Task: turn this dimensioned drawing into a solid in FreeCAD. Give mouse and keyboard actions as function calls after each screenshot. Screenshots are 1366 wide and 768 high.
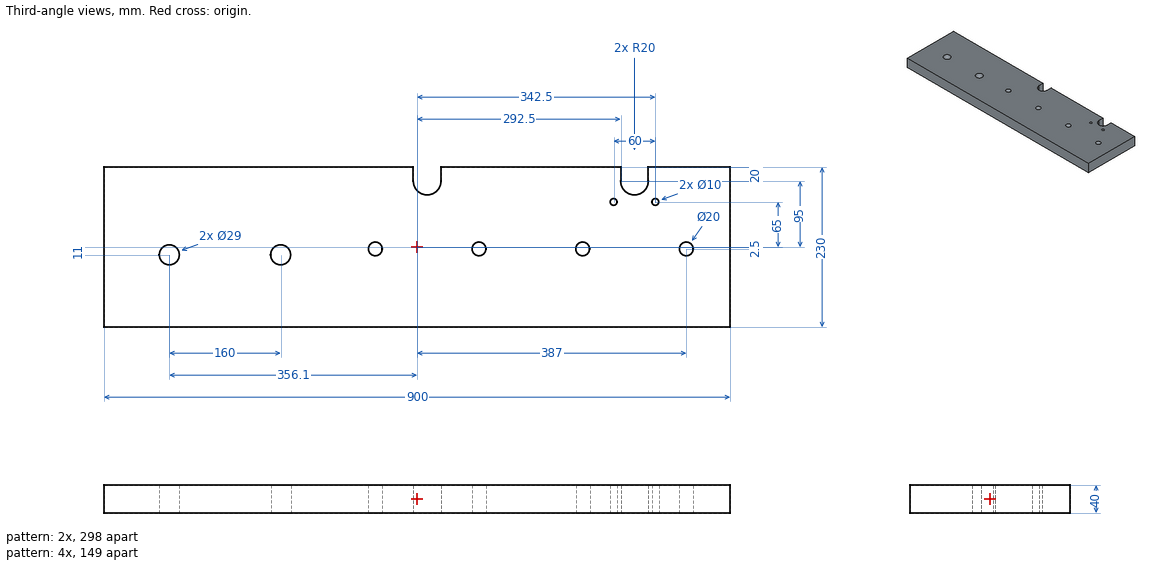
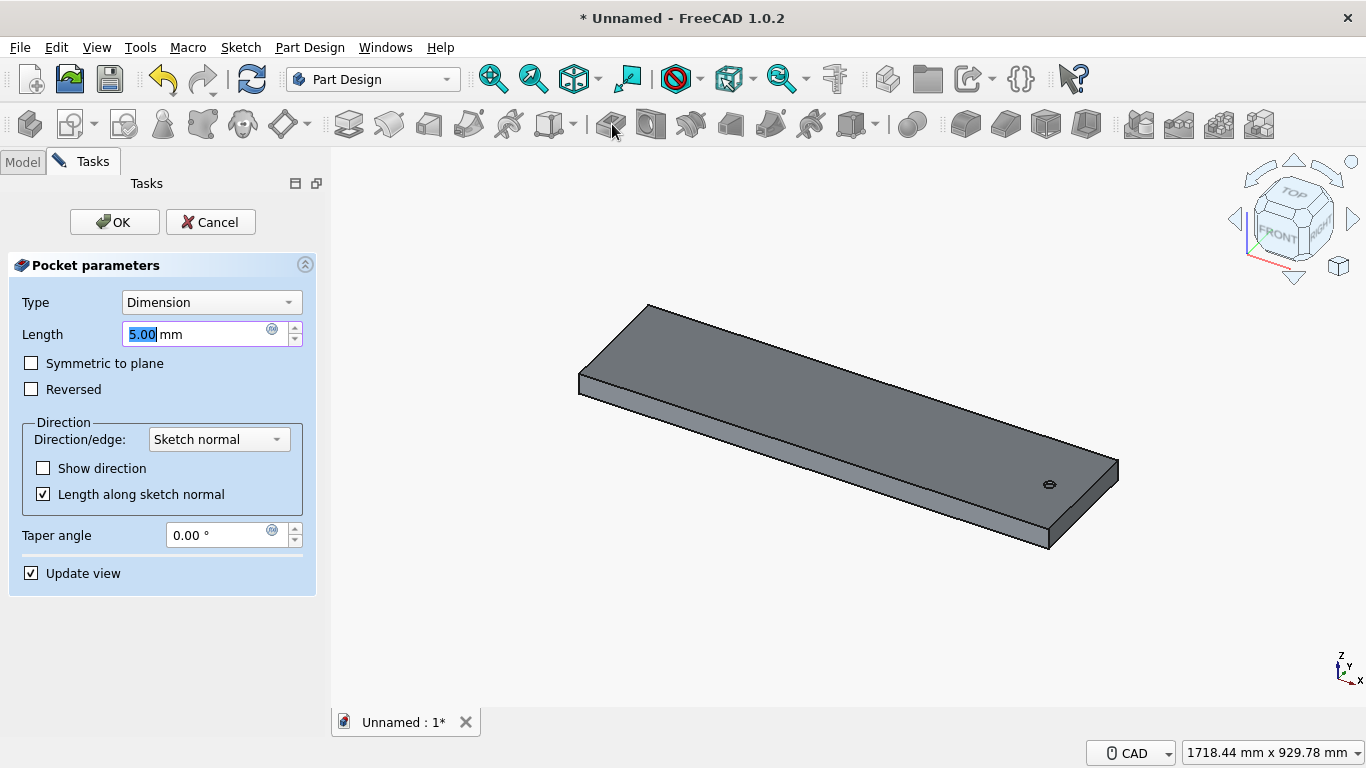
click(212, 302)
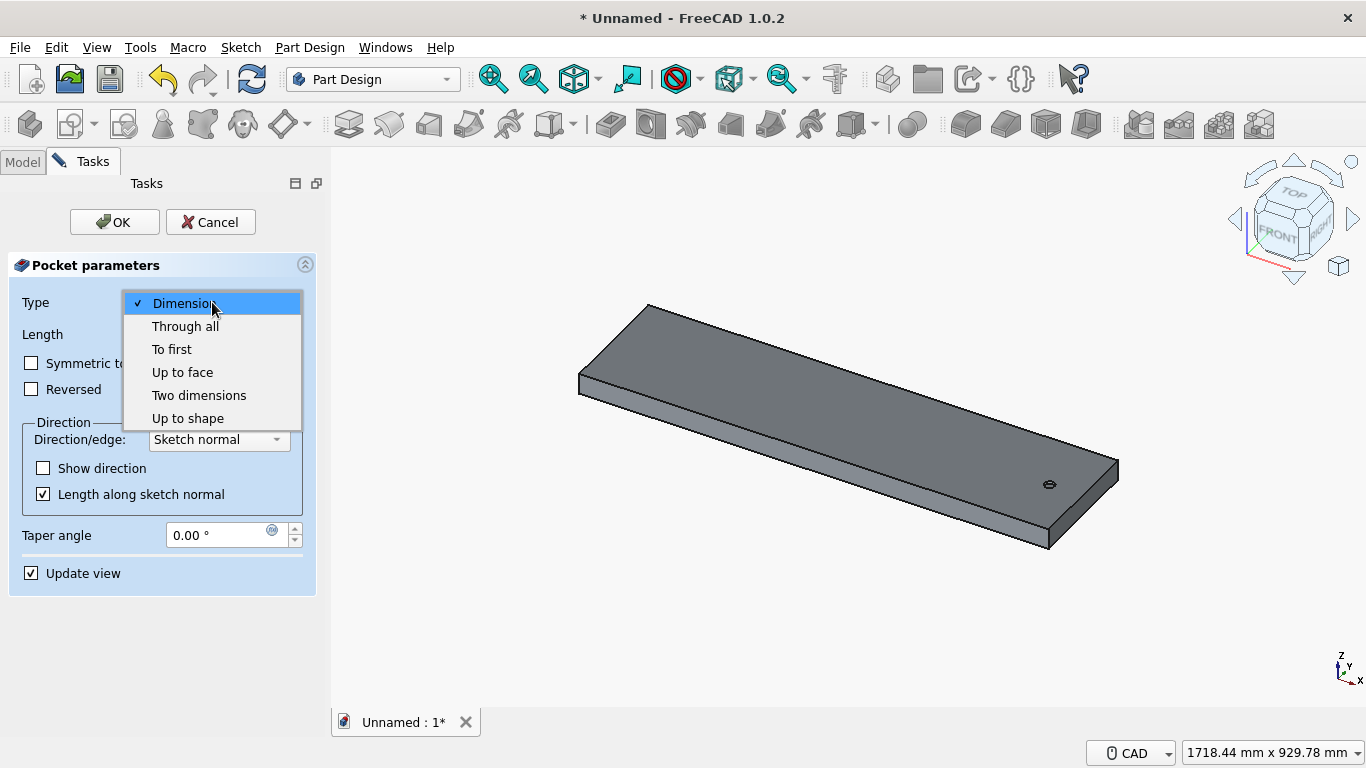
click(212, 326)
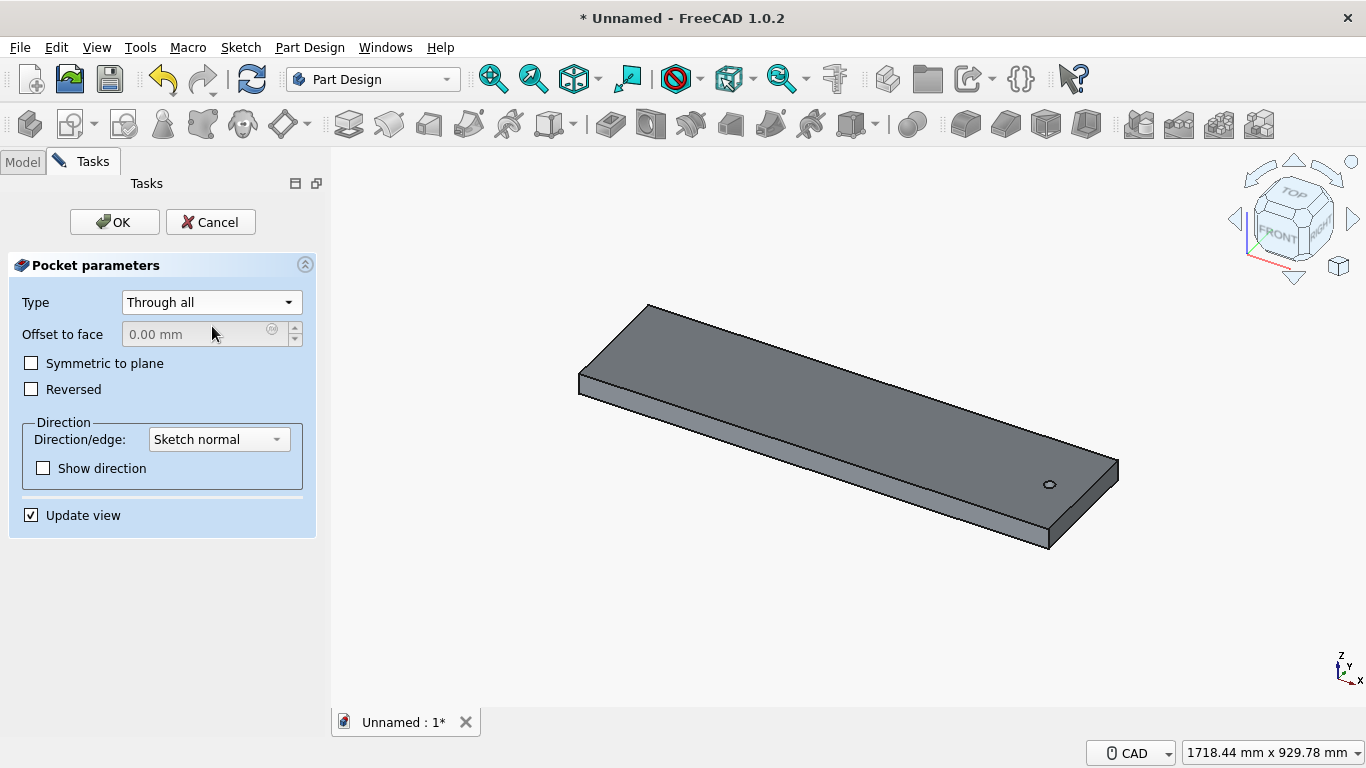
click(115, 222)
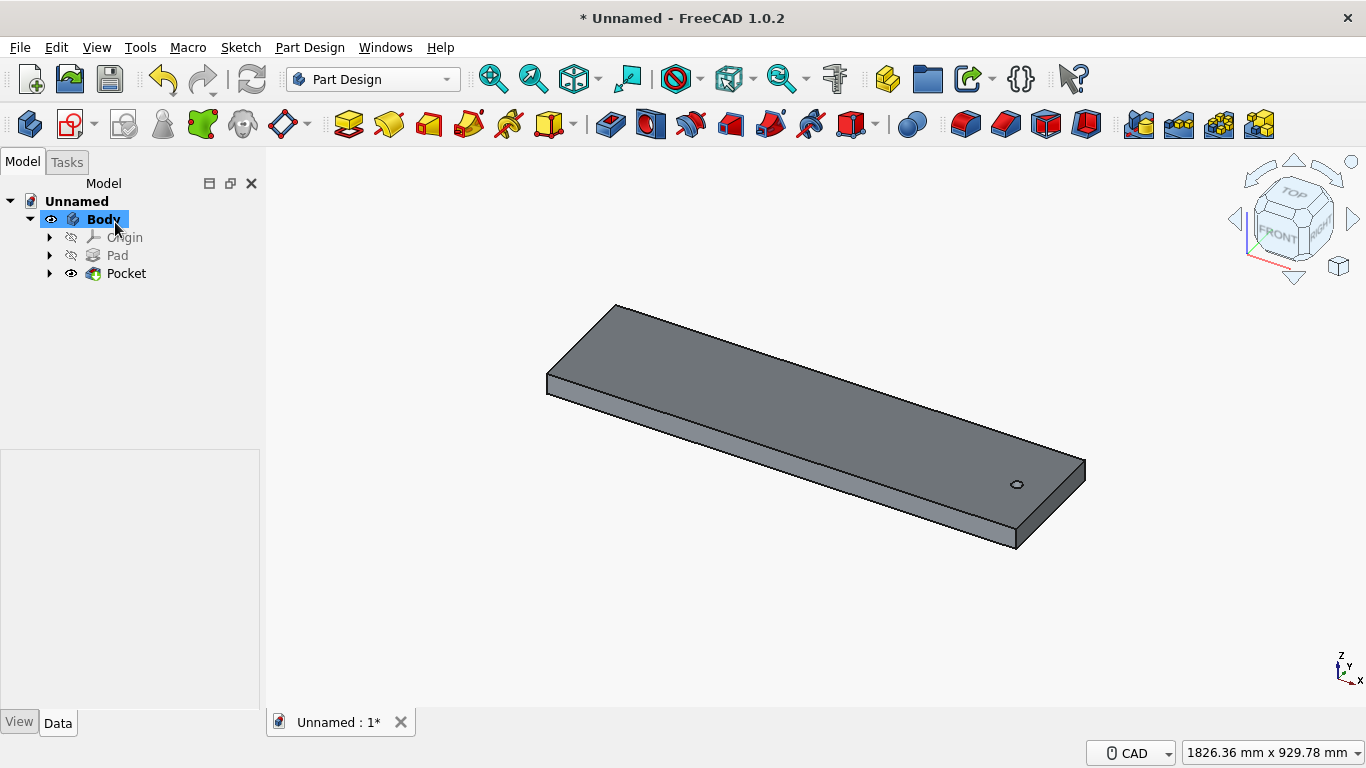
click(950, 461)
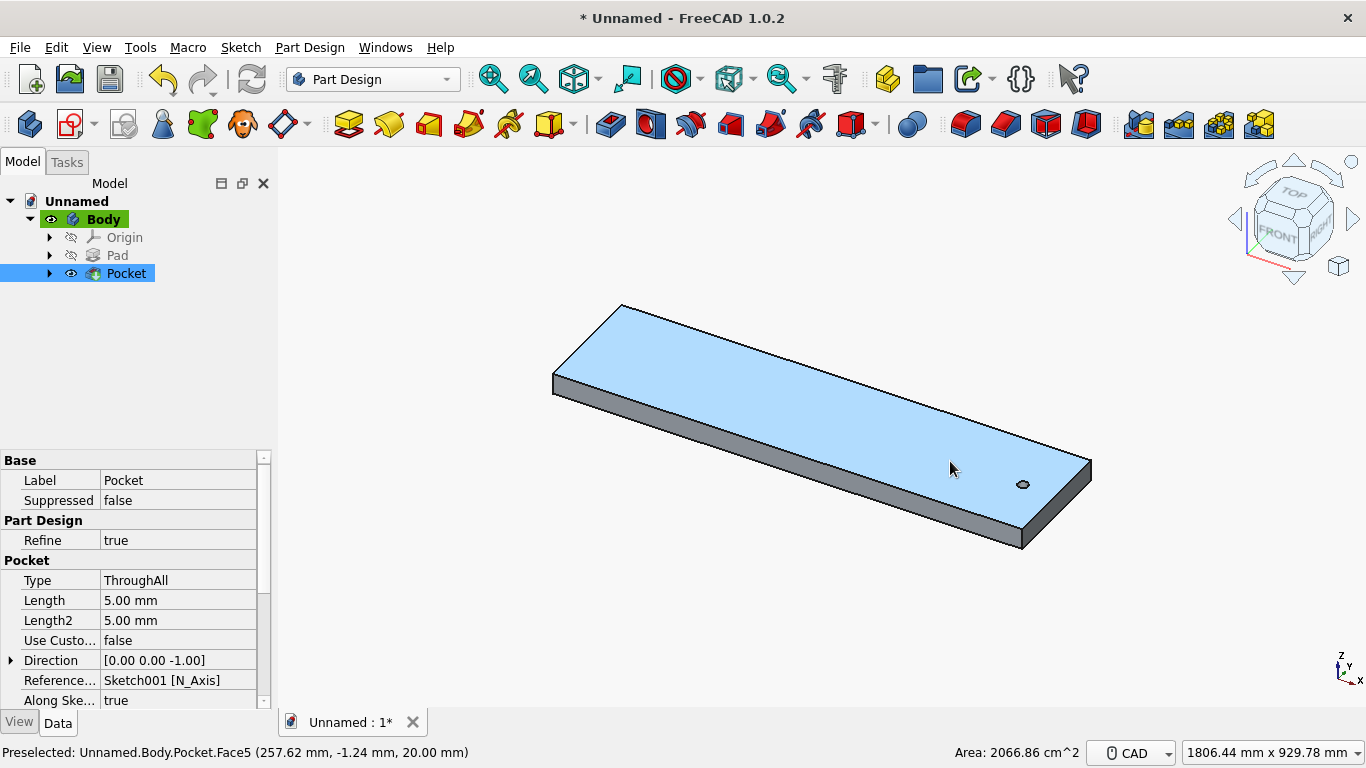
click(70, 124)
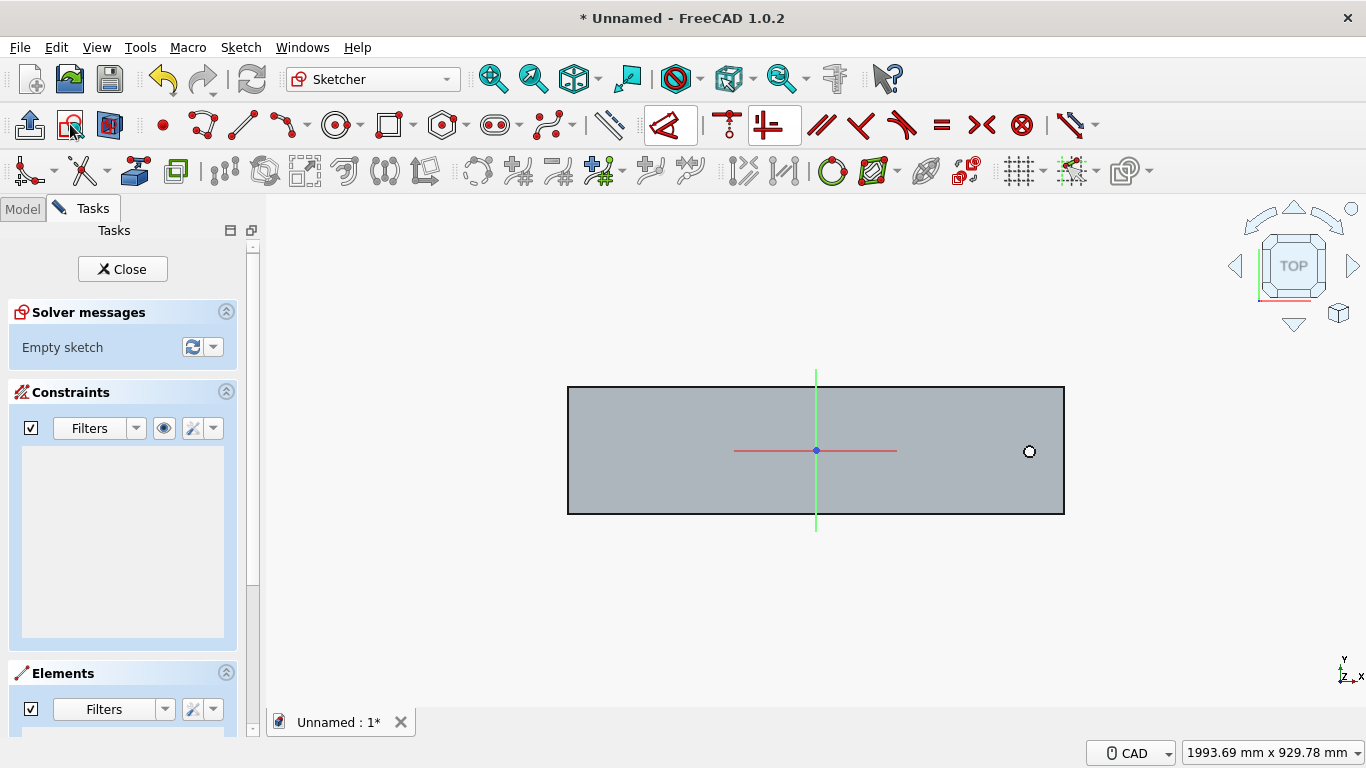
scroll(1018, 385, up, 11)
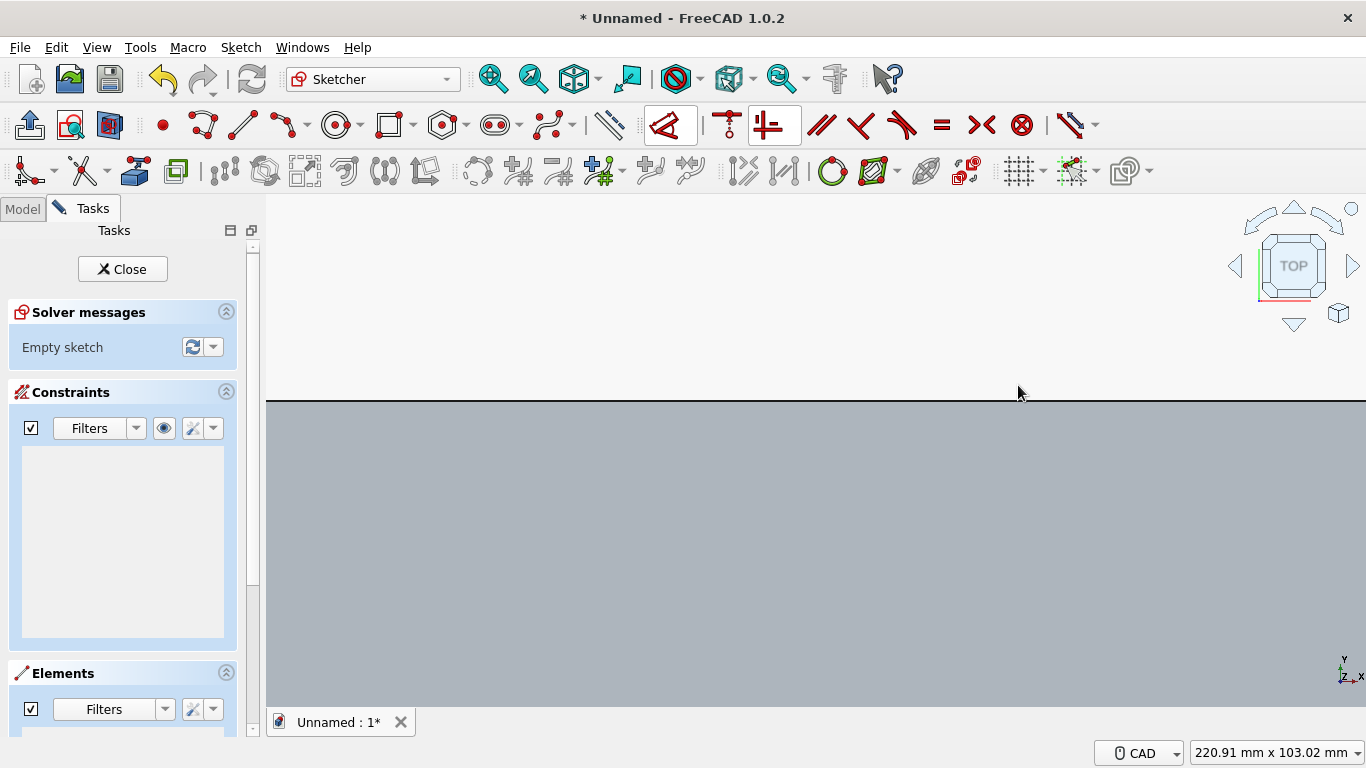
key(g)
key(s)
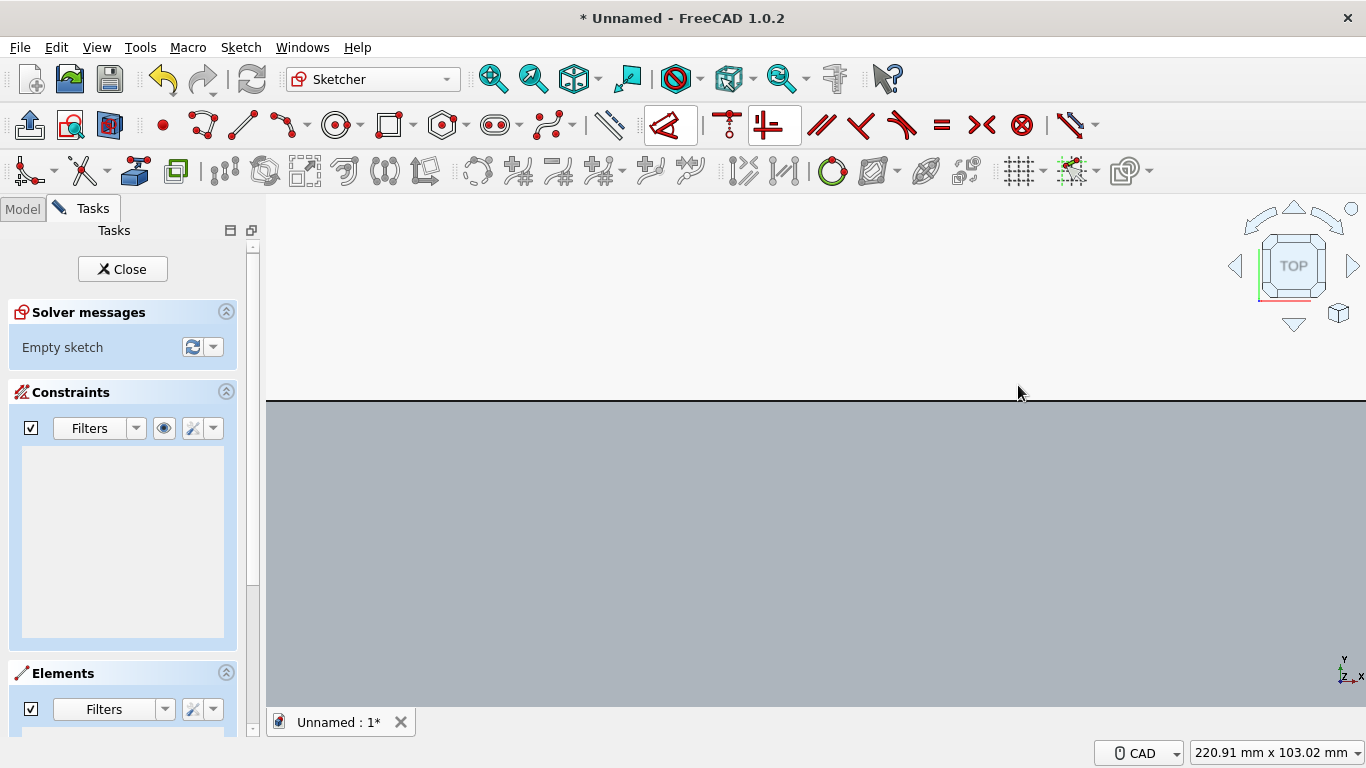
click(746, 500)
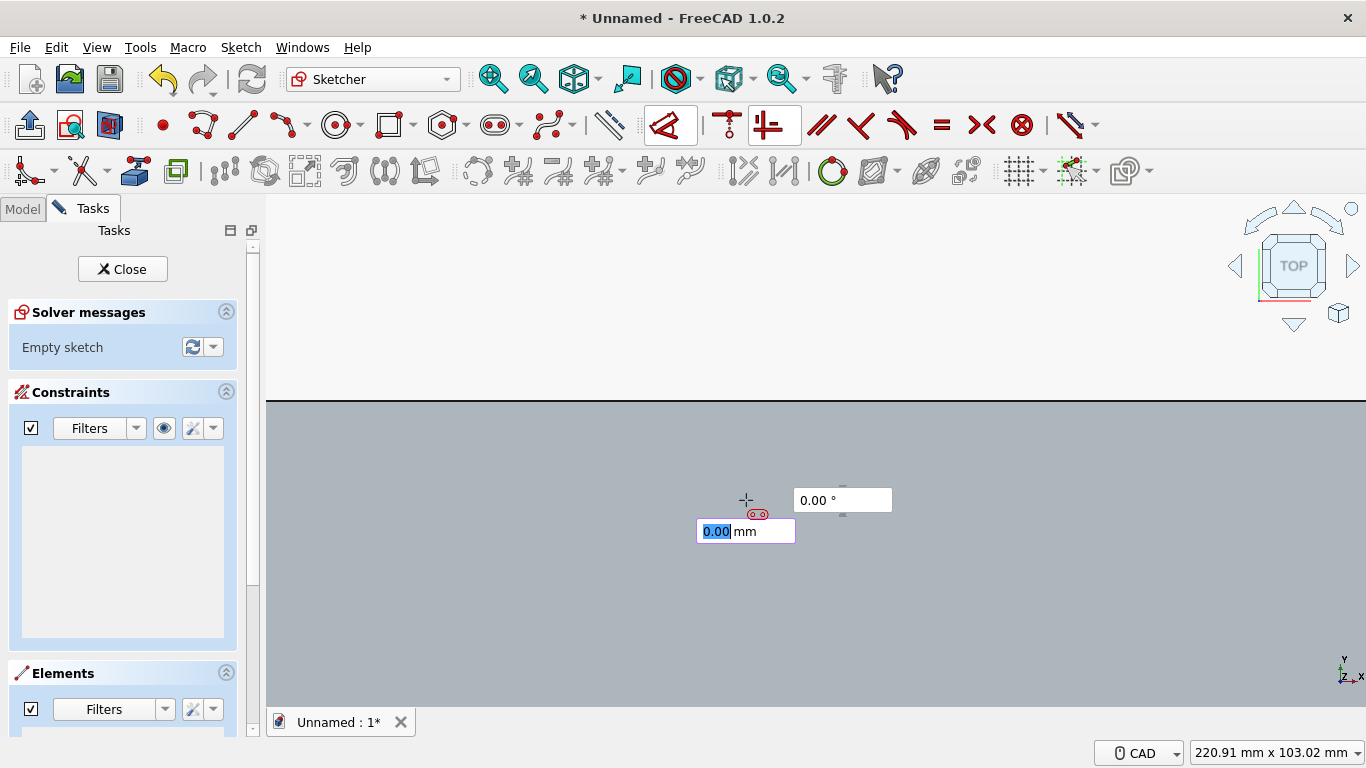
click(746, 401)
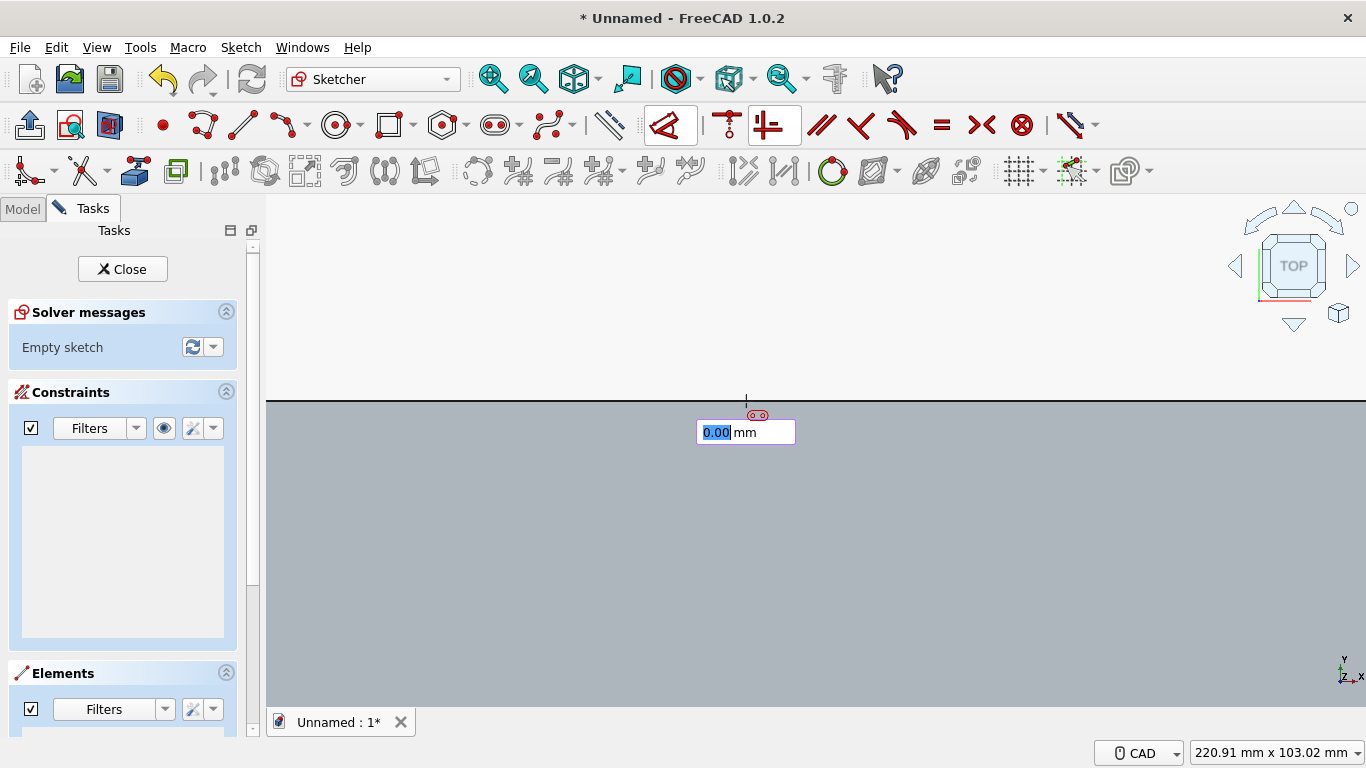
click(845, 450)
key(Escape)